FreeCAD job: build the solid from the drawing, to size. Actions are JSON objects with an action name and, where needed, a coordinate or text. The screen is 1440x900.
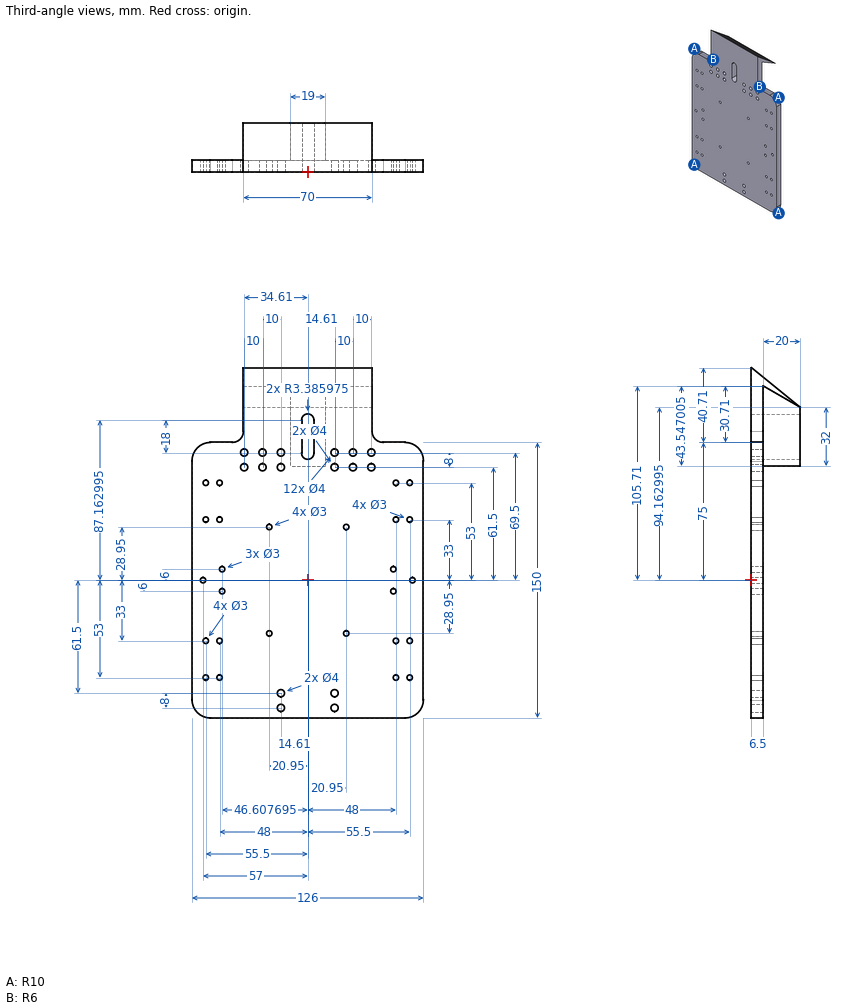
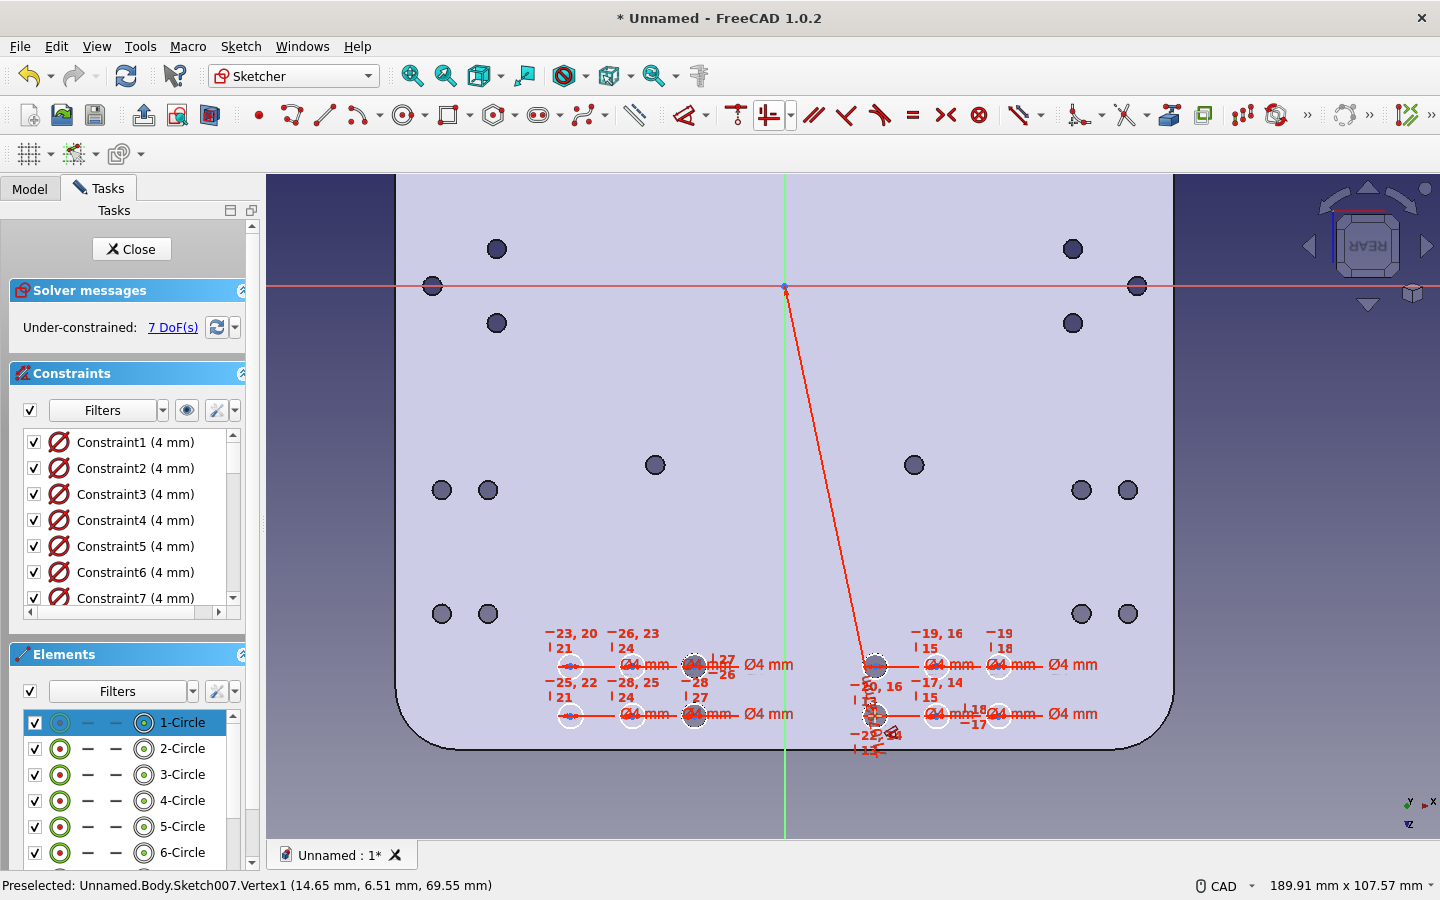
{"action": "left_click", "coordinate": [875, 667]}
{"action": "left_click", "coordinate": [909, 691]}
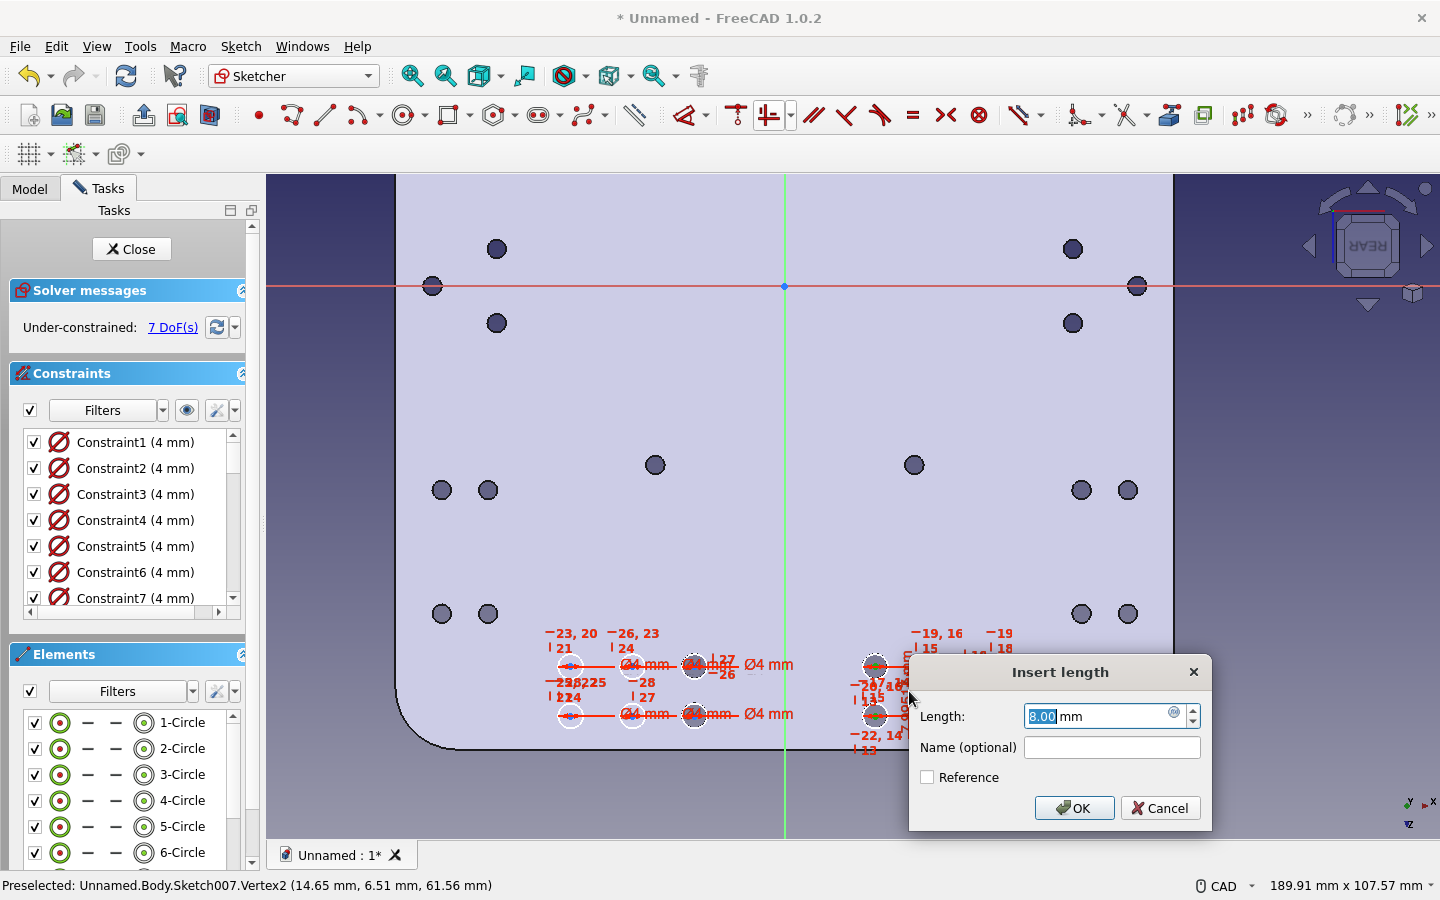
{"action": "type", "text": "8"}
{"action": "key", "text": "Return"}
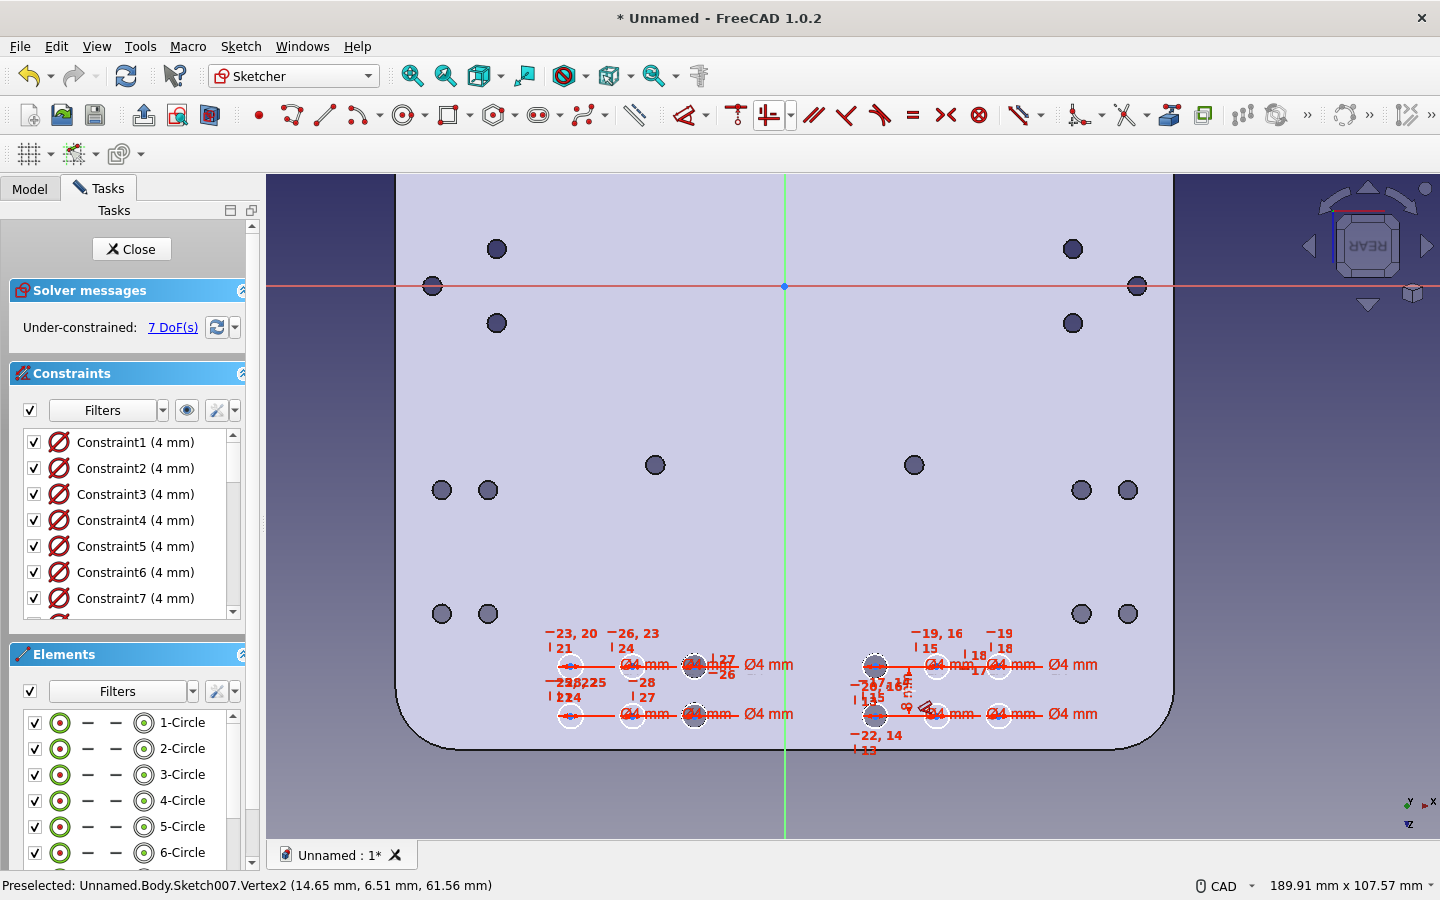
{"action": "left_click", "coordinate": [875, 716]}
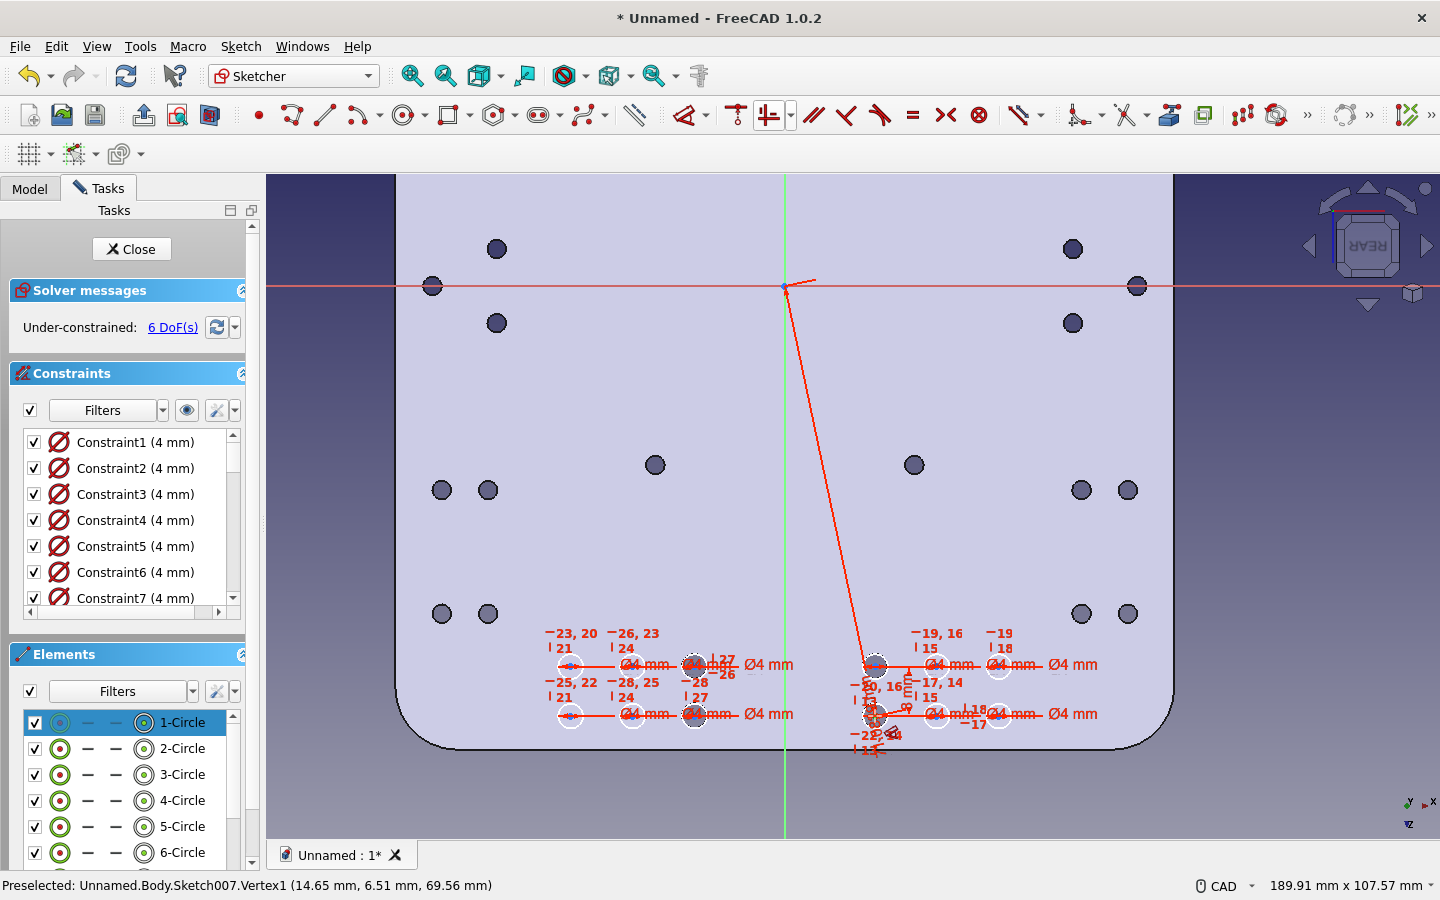
{"action": "left_click", "coordinate": [937, 716]}
{"action": "left_click", "coordinate": [906, 750]}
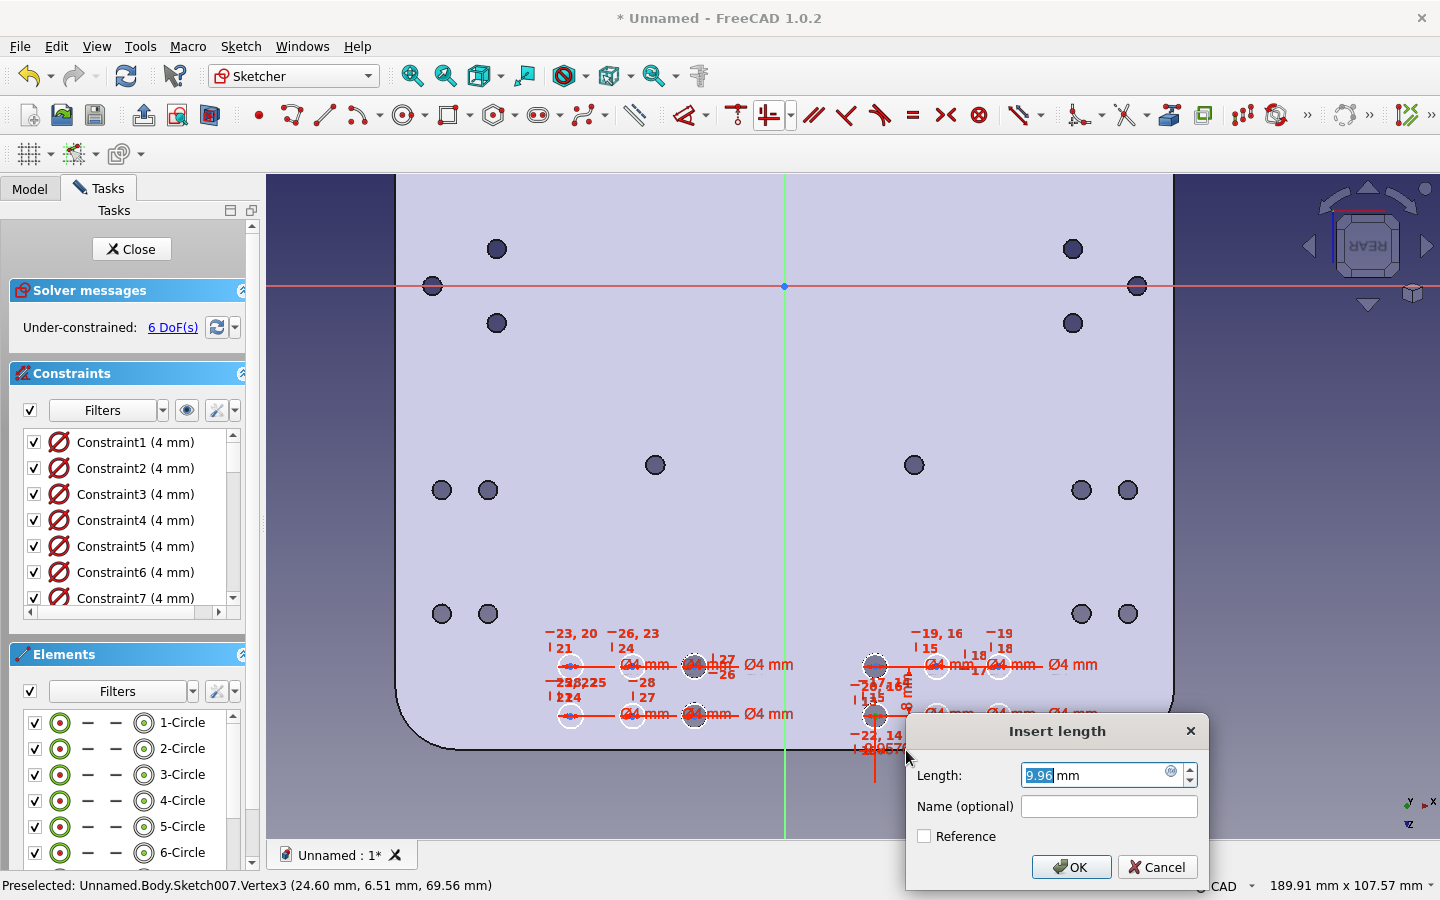
{"action": "type", "text": "10"}
{"action": "key", "text": "Return"}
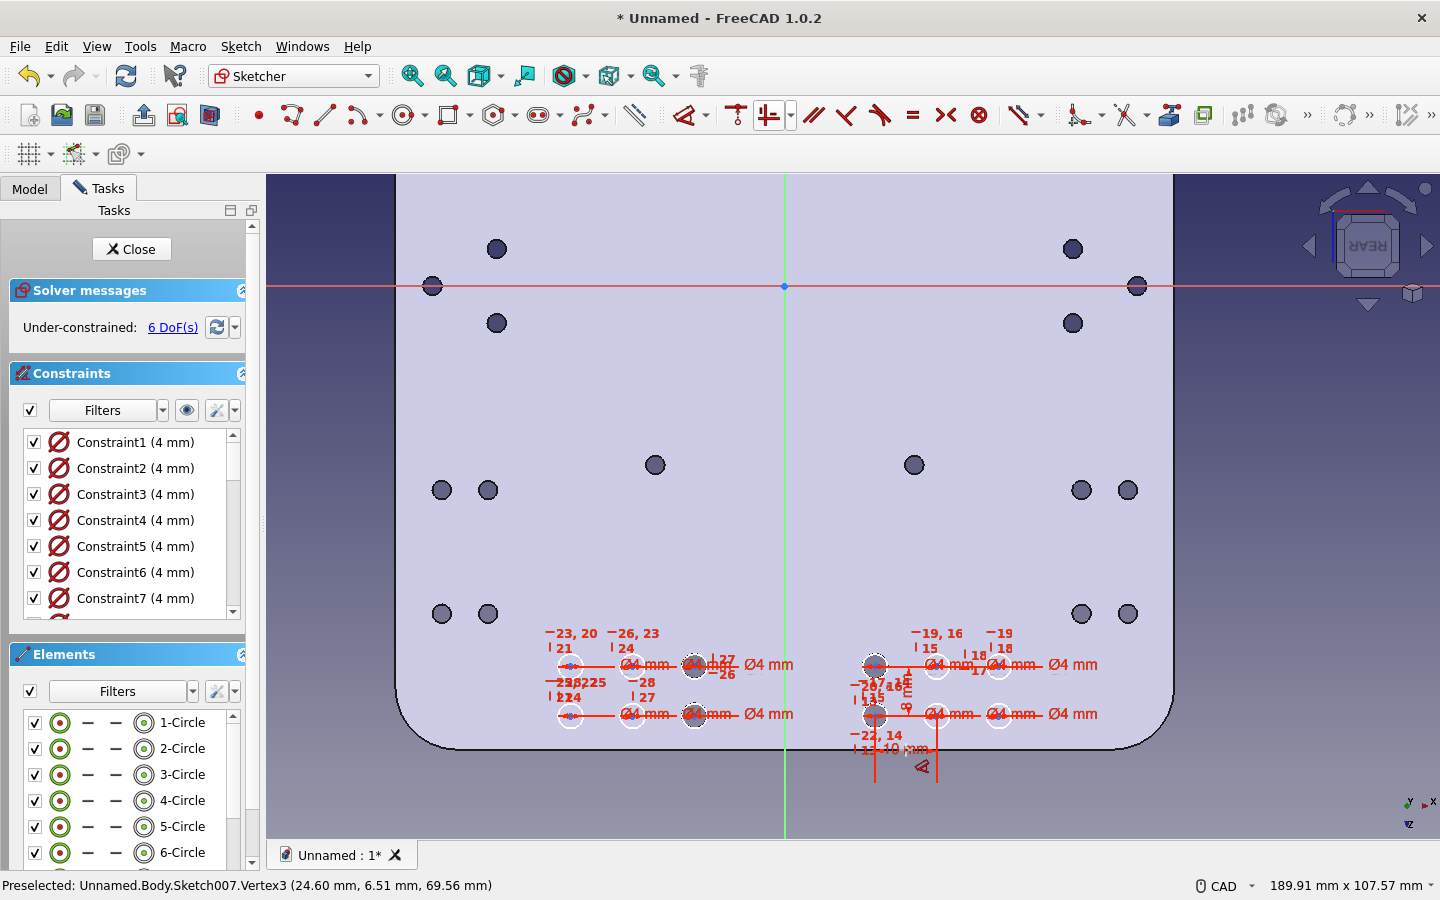
{"action": "left_click", "coordinate": [937, 716]}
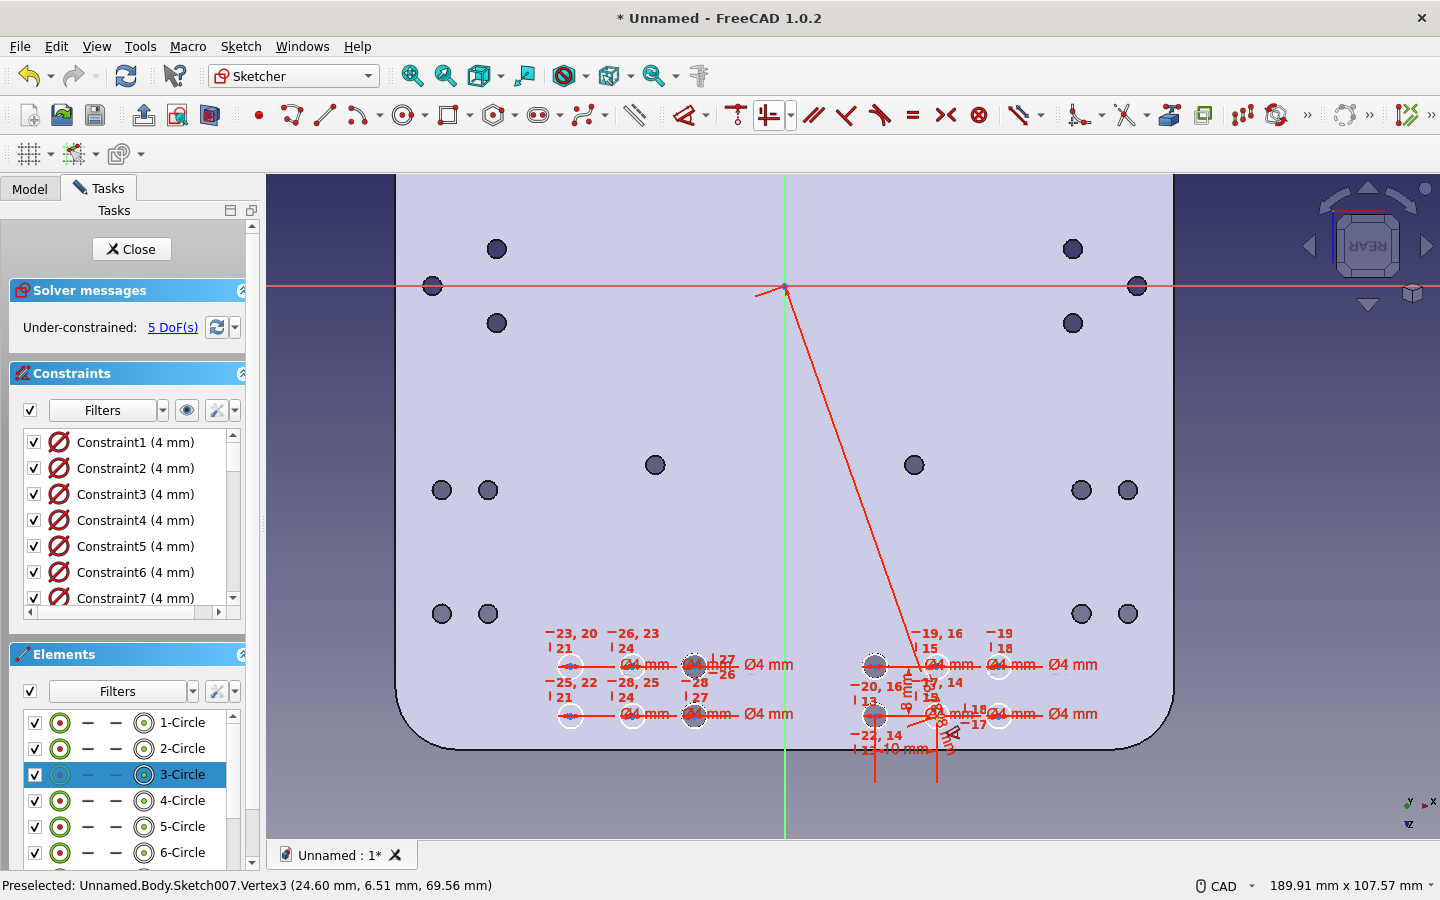
{"action": "left_click", "coordinate": [999, 716]}
{"action": "left_click", "coordinate": [982, 750]}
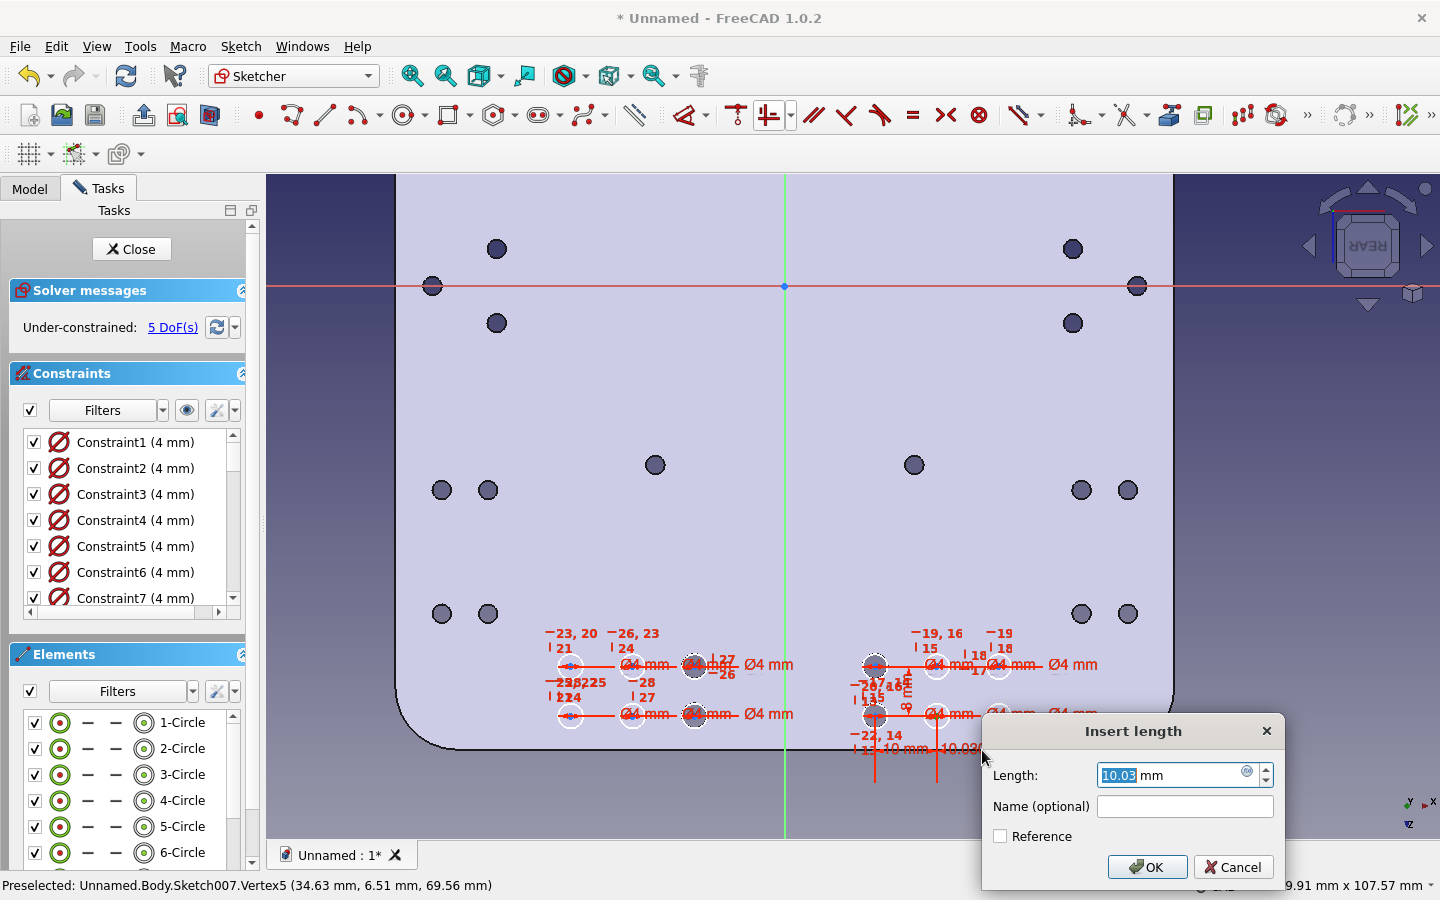
{"action": "type", "text": "10"}
{"action": "key", "text": "Return"}